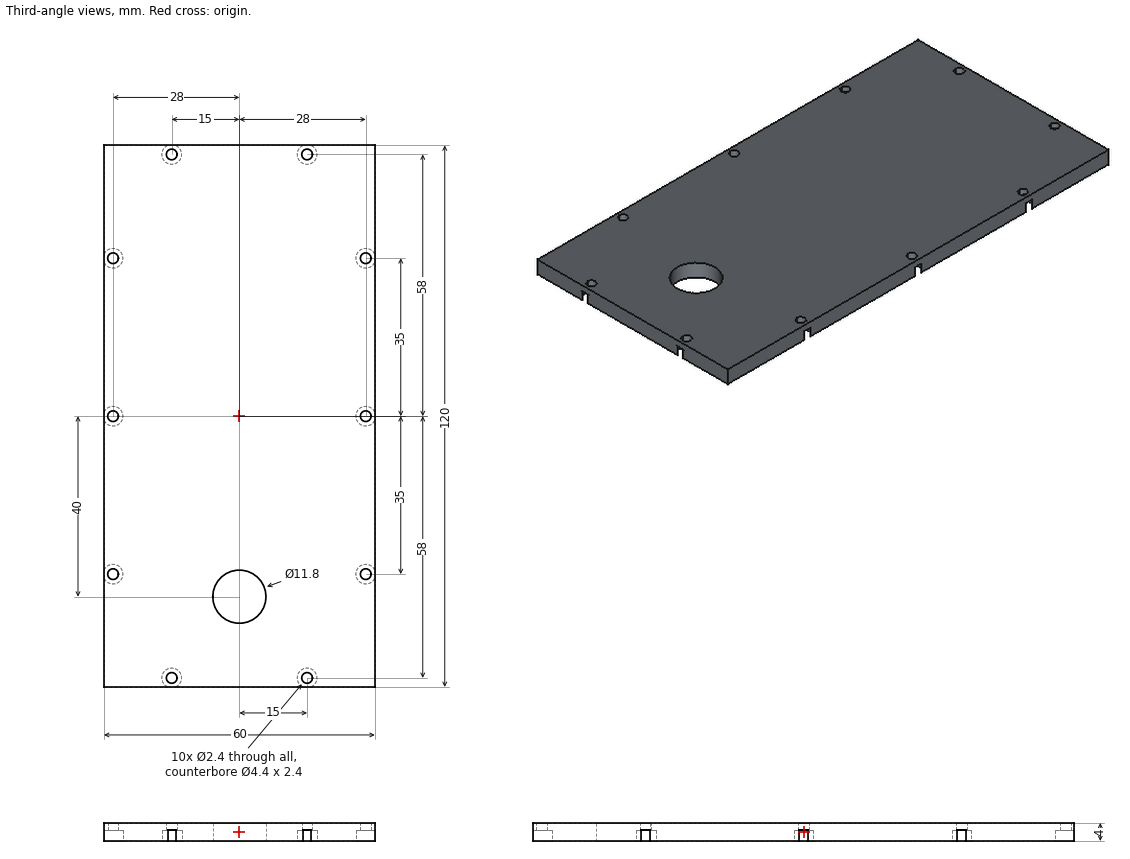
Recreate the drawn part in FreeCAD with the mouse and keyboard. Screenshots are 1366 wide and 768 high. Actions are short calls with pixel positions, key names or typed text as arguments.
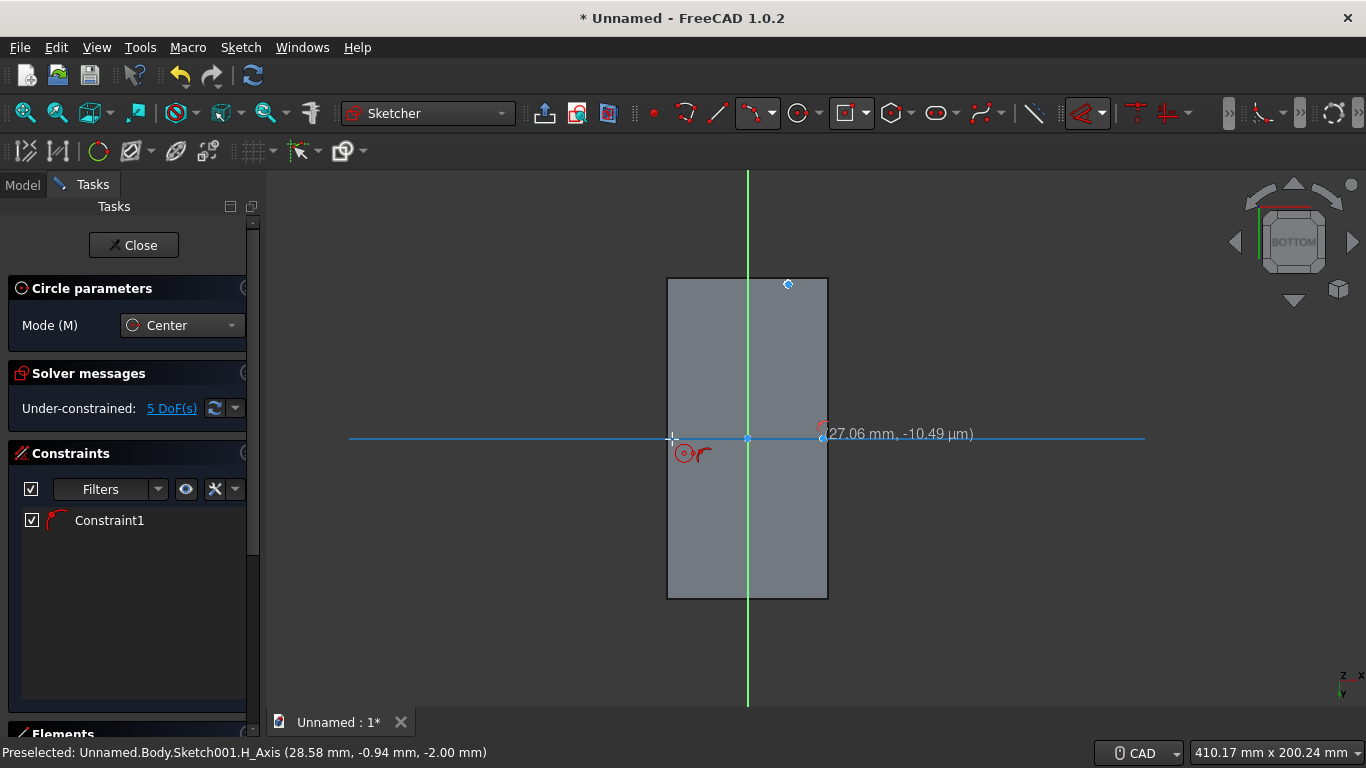
click(672, 439)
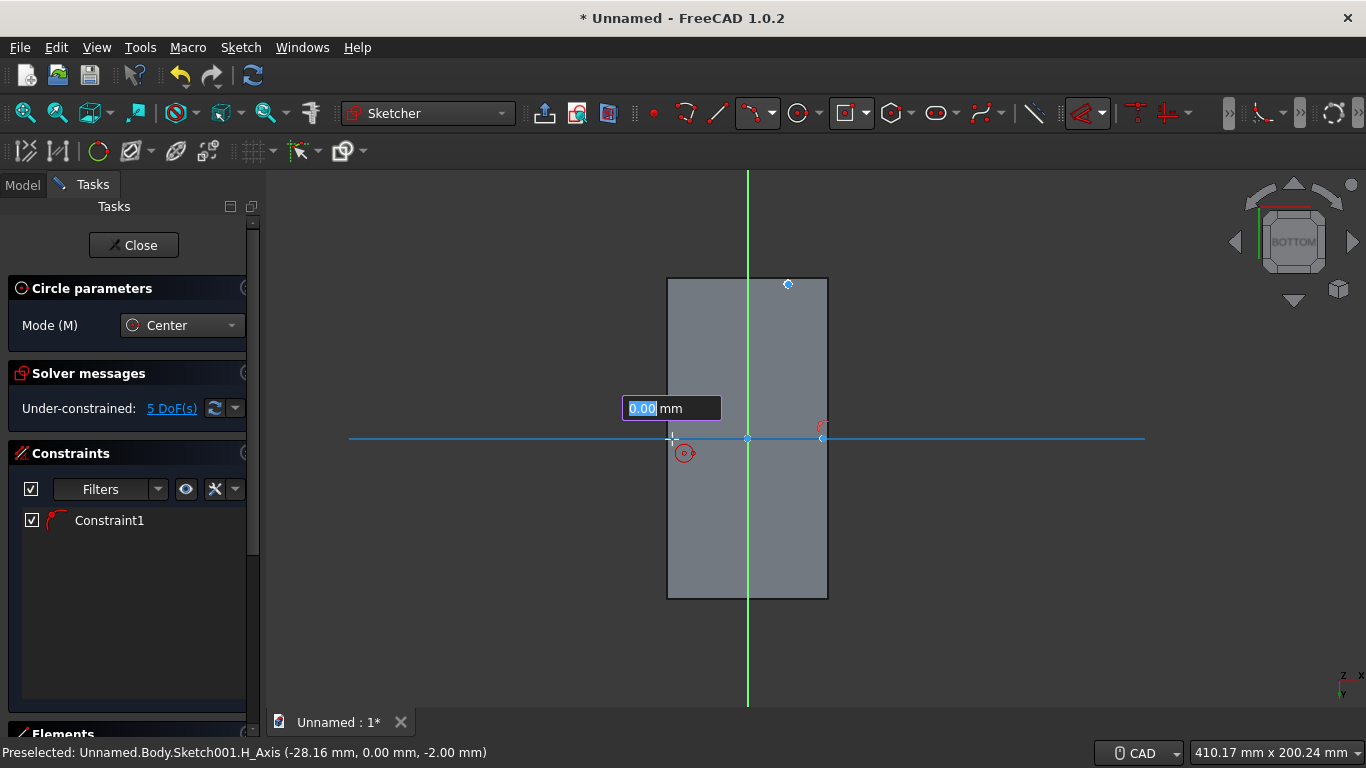
scroll(674, 436, up, 9)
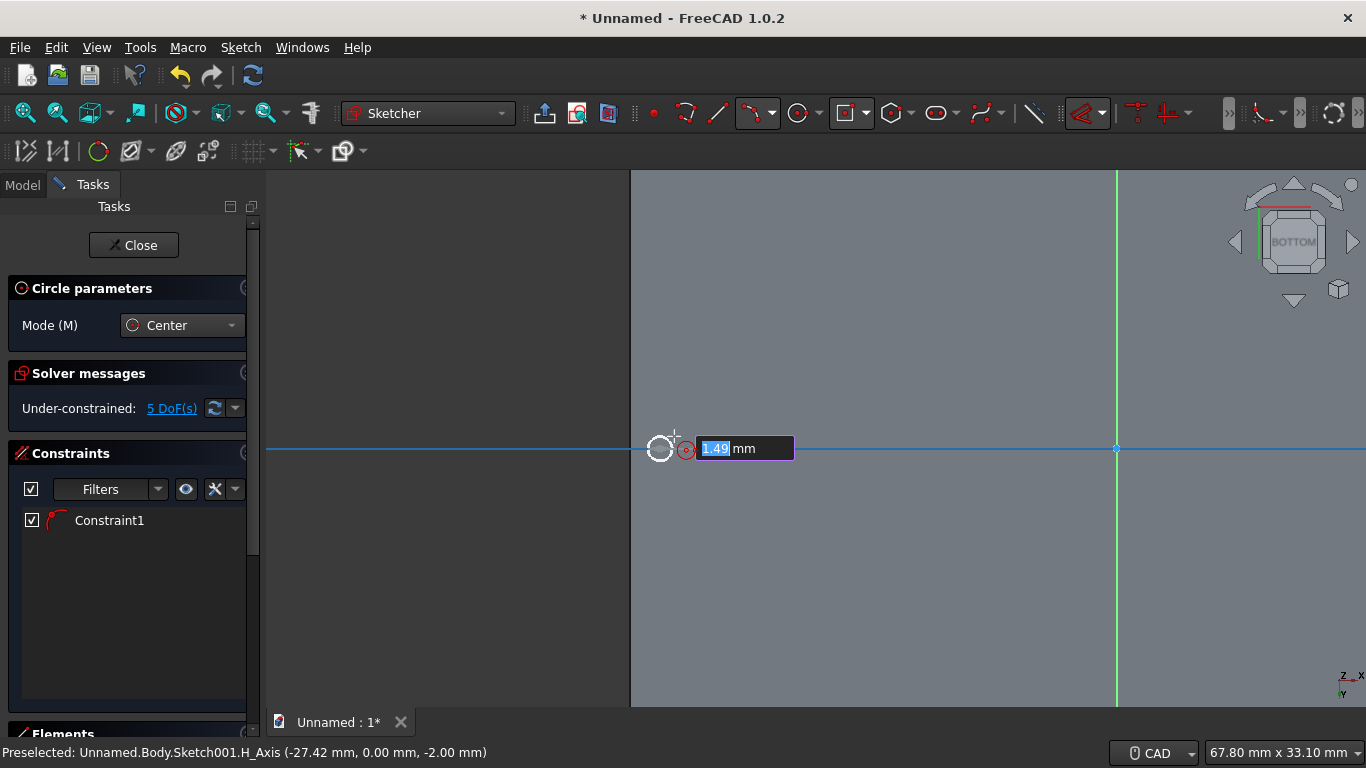
click(669, 431)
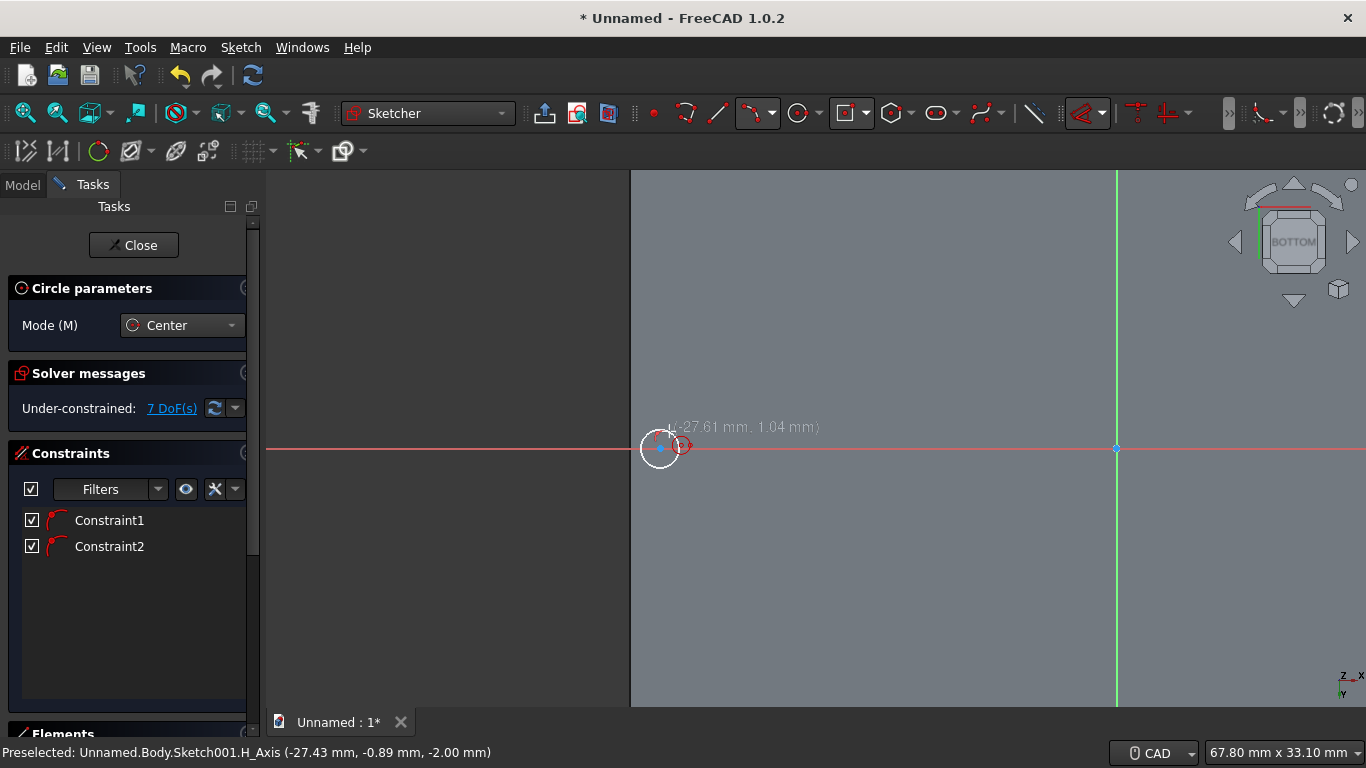
scroll(674, 436, down, 9)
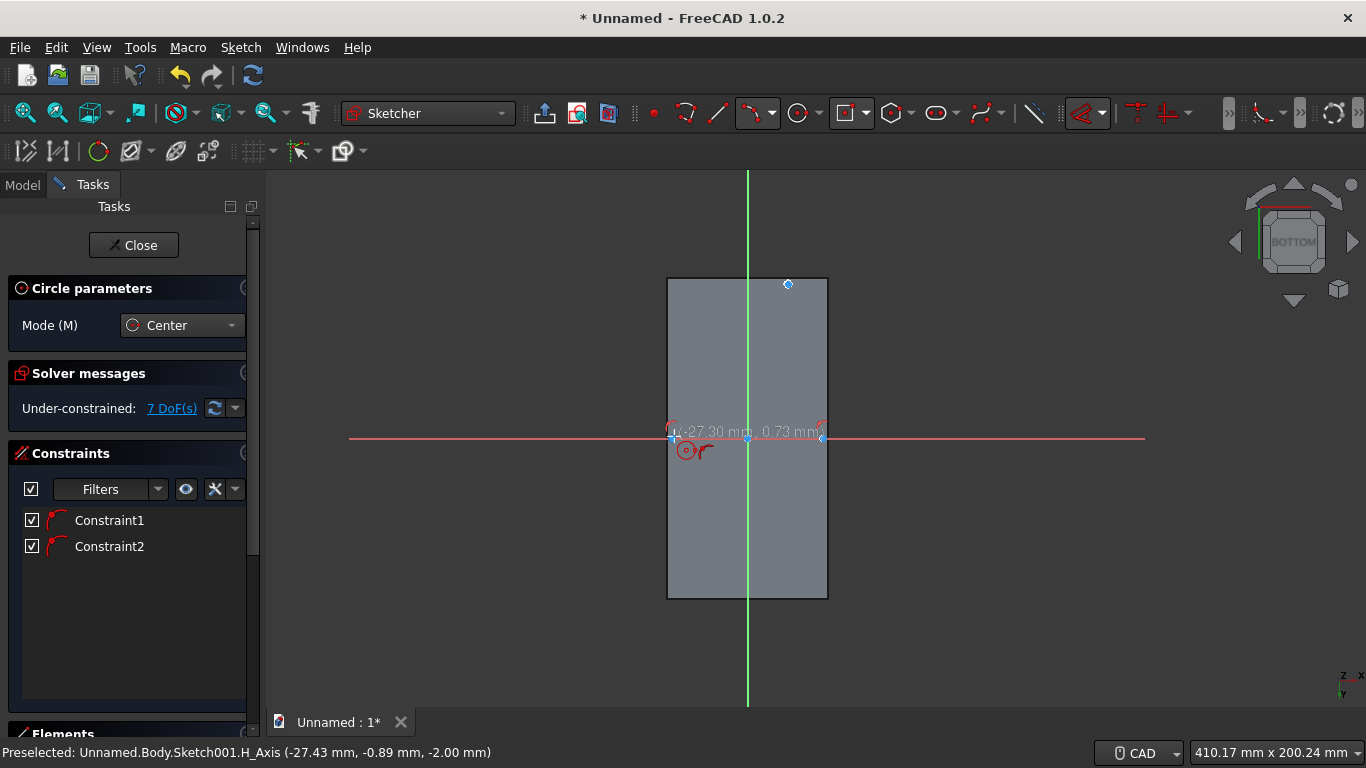
scroll(788, 594, up, 10)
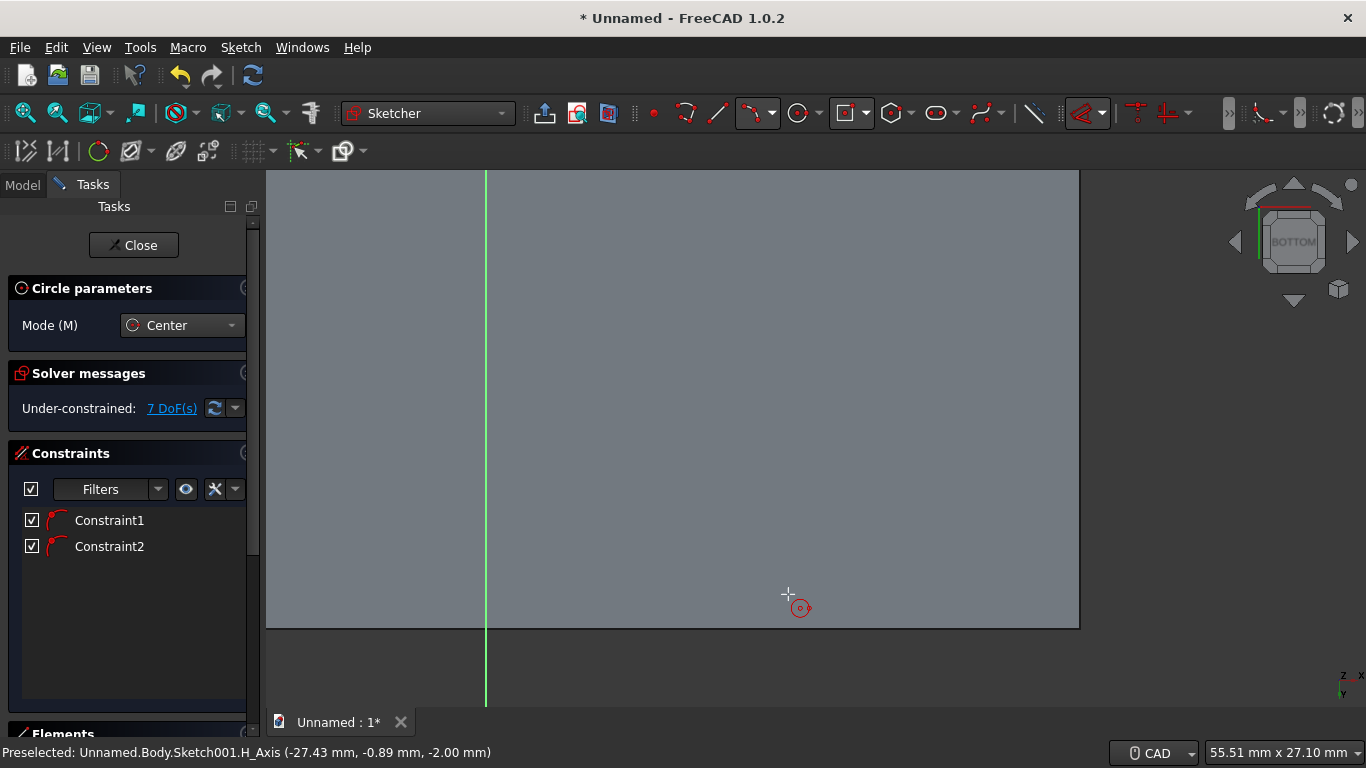
scroll(788, 595, down, 10)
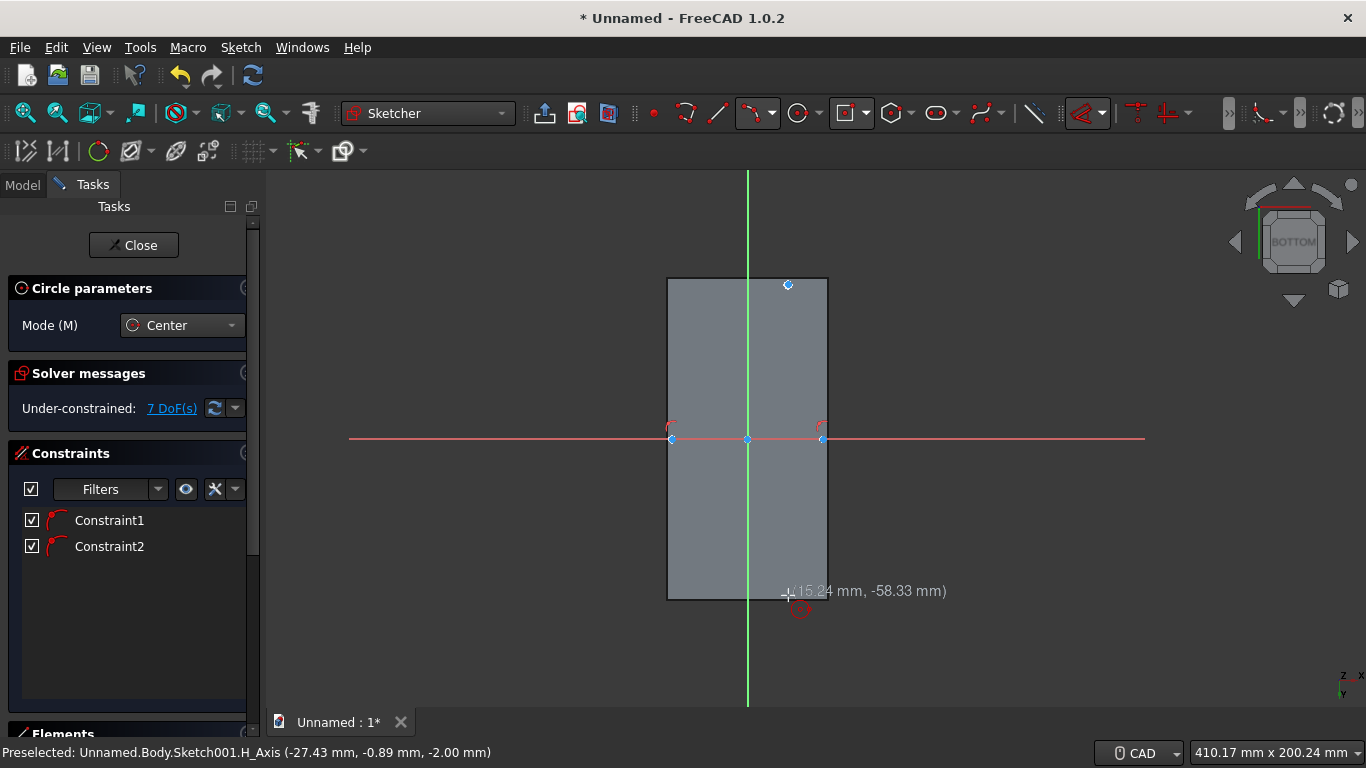
click(788, 595)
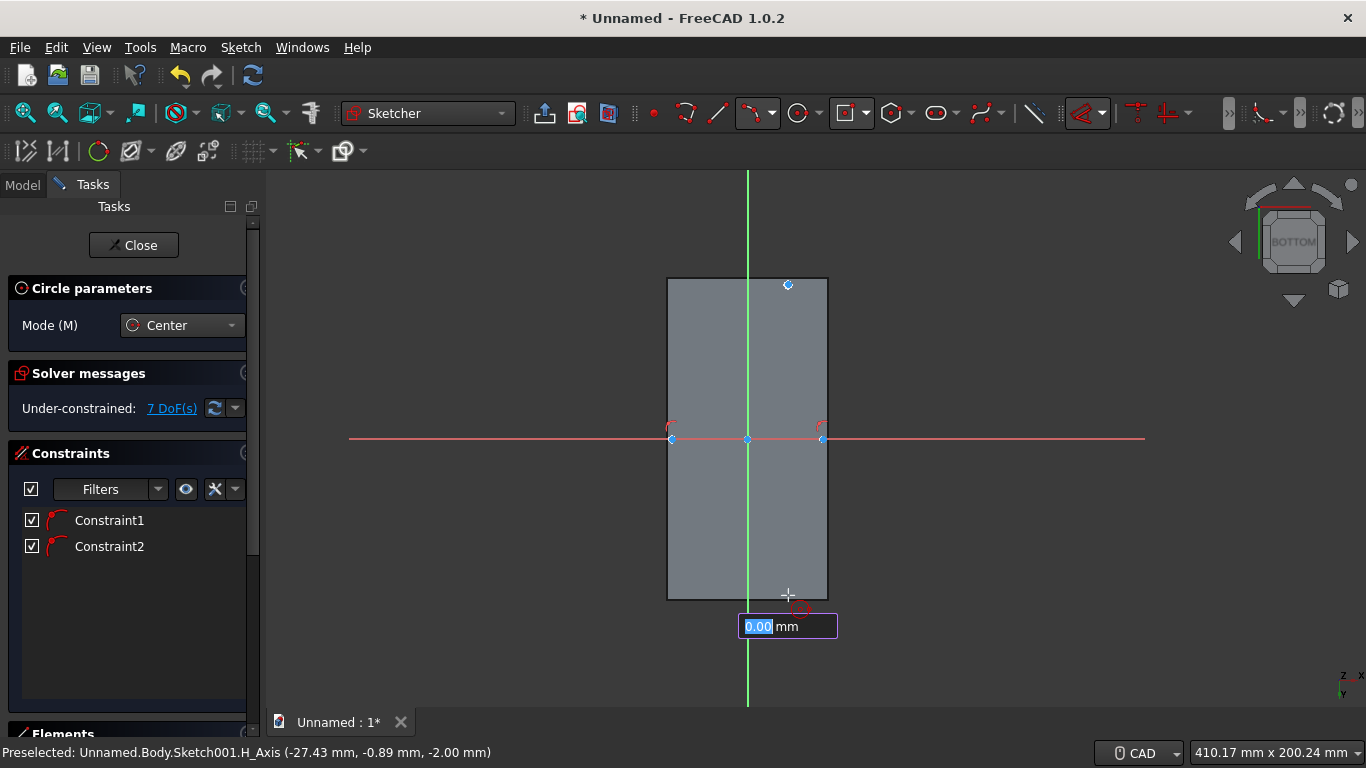
scroll(790, 593, up, 8)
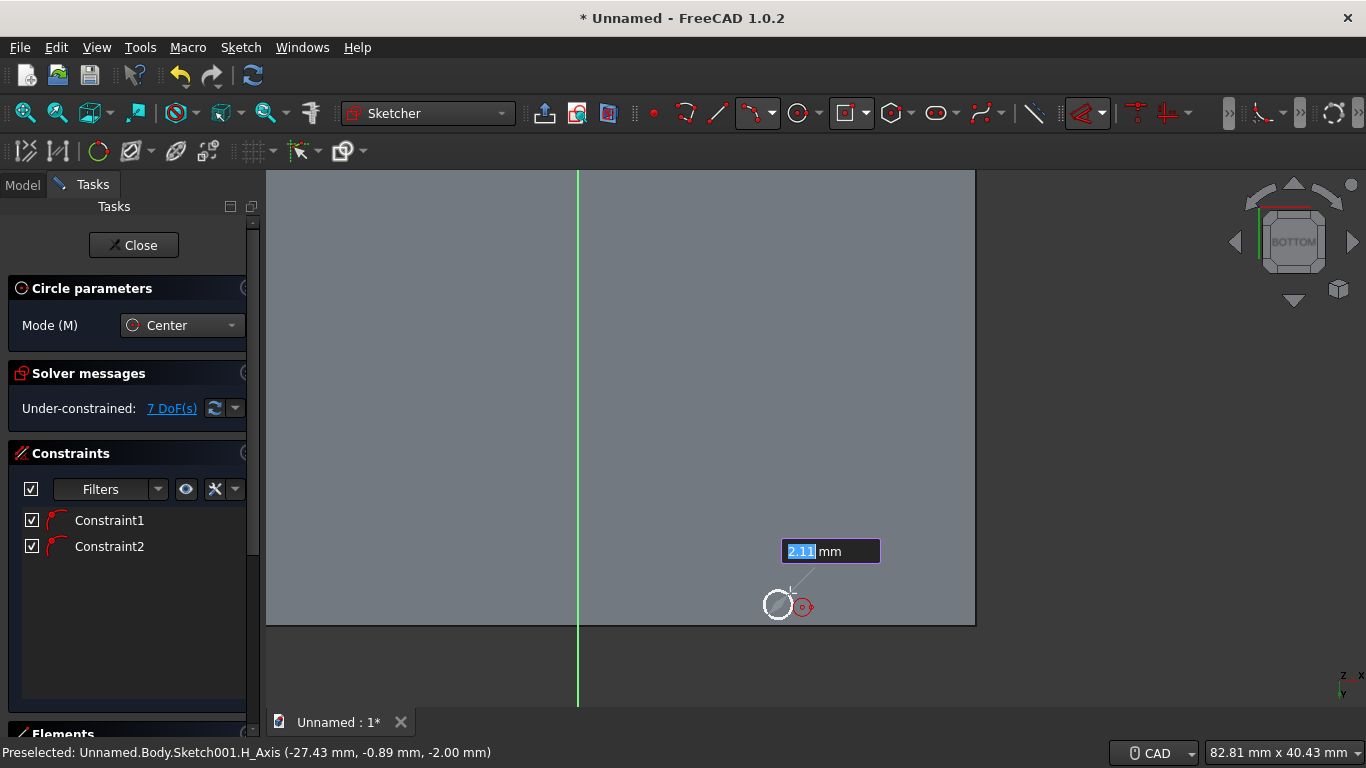
click(788, 588)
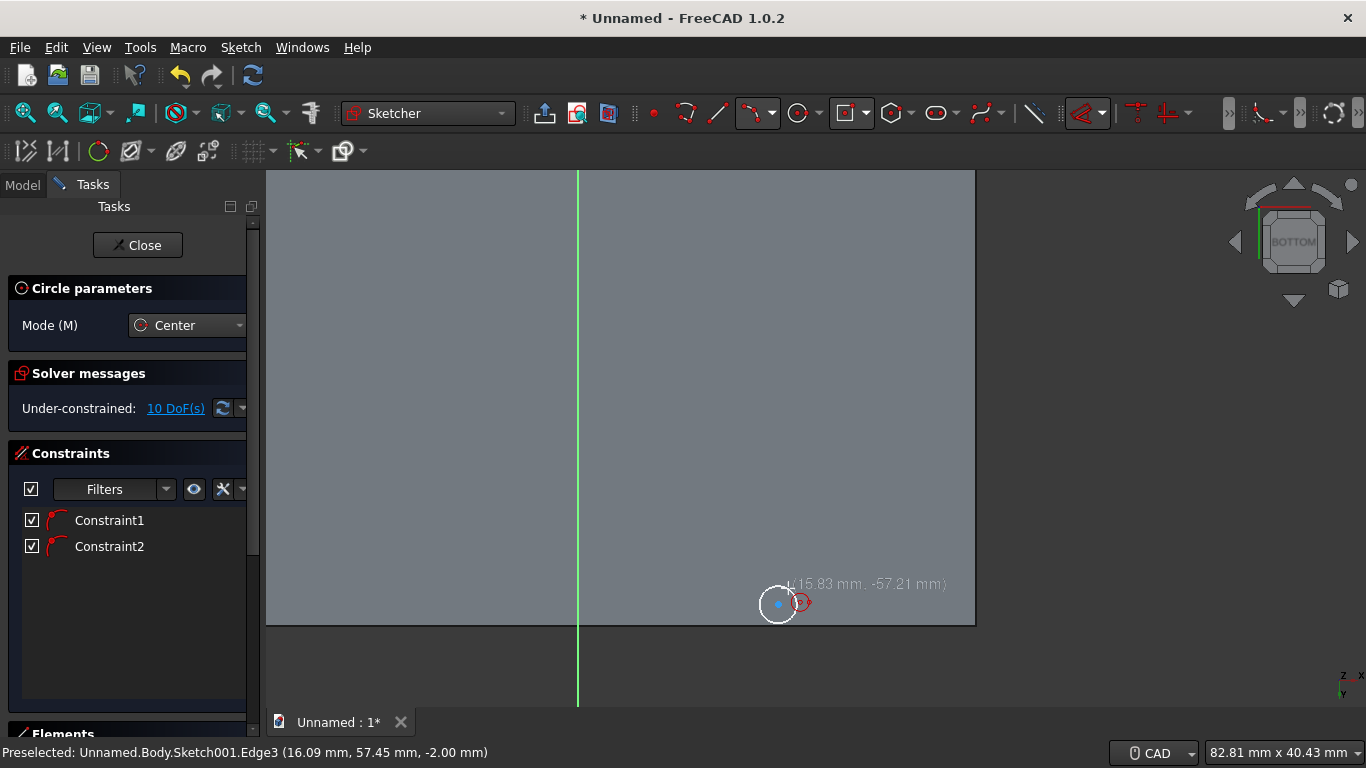
scroll(379, 599, up, 2)